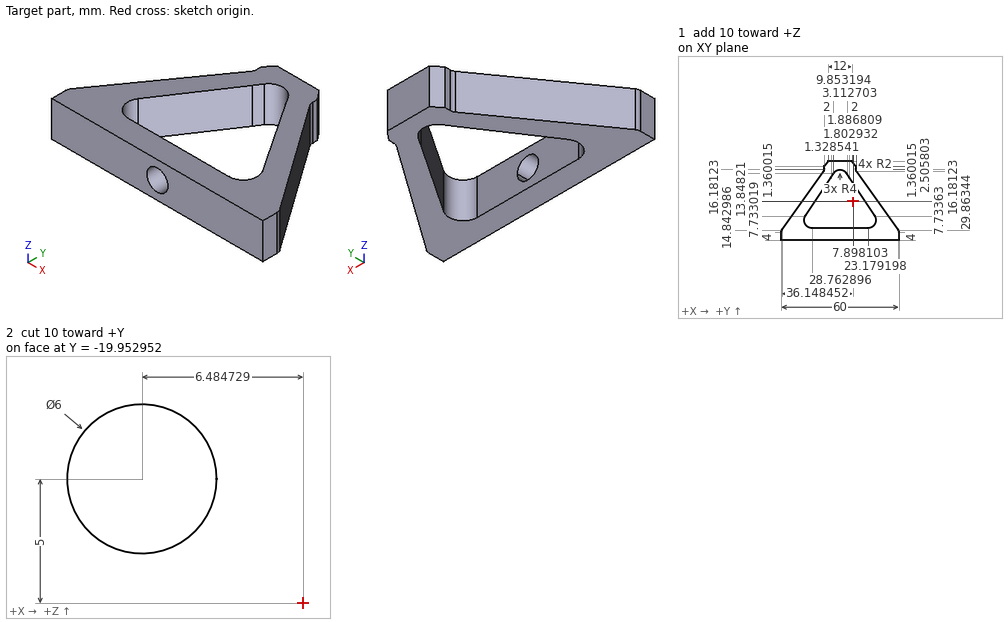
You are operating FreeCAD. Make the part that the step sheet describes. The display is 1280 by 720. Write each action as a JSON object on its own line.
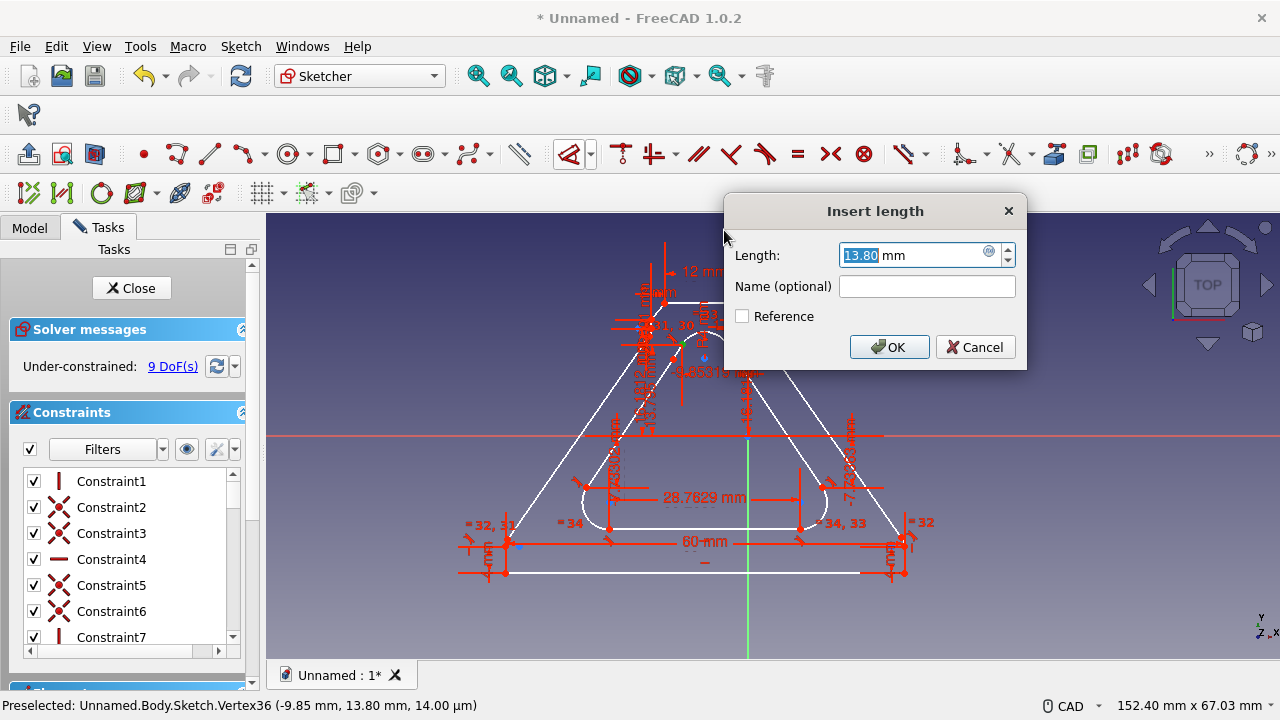
{"action": "type", "text": "13.84821"}
{"action": "key", "text": "Return"}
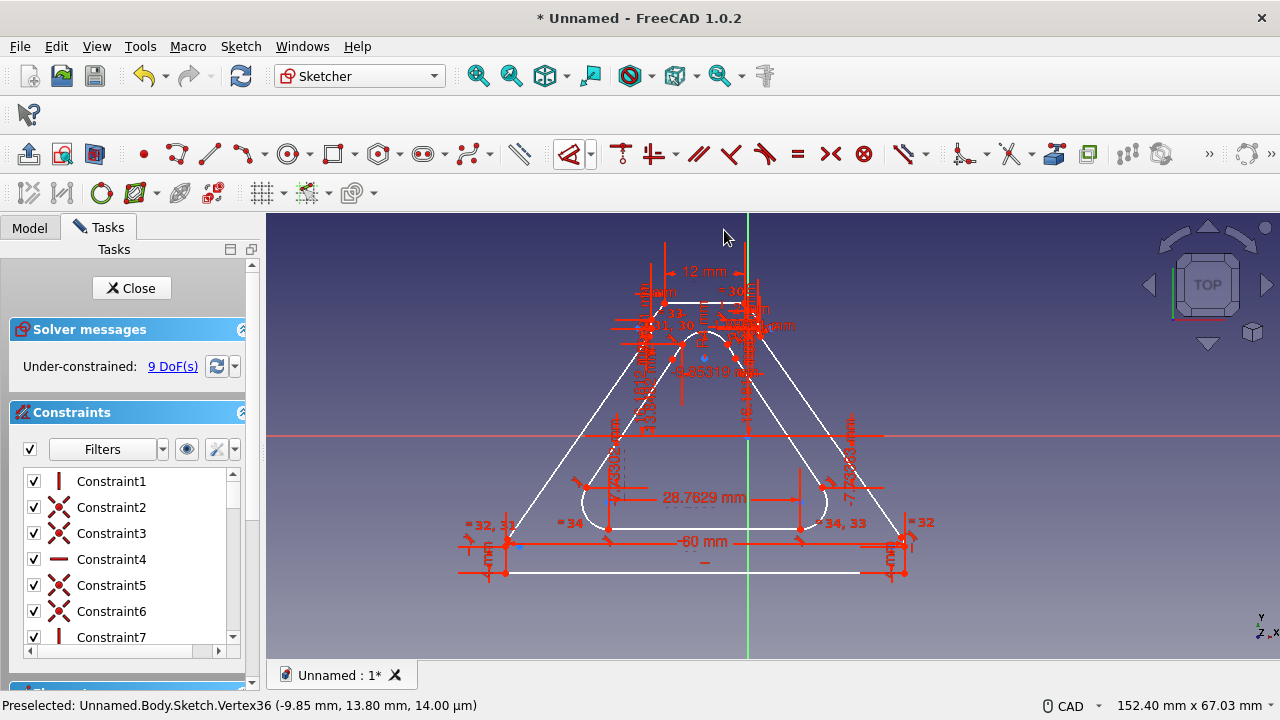
{"action": "scroll", "coordinate": [728, 345], "scroll_direction": "up", "scroll_amount": 4}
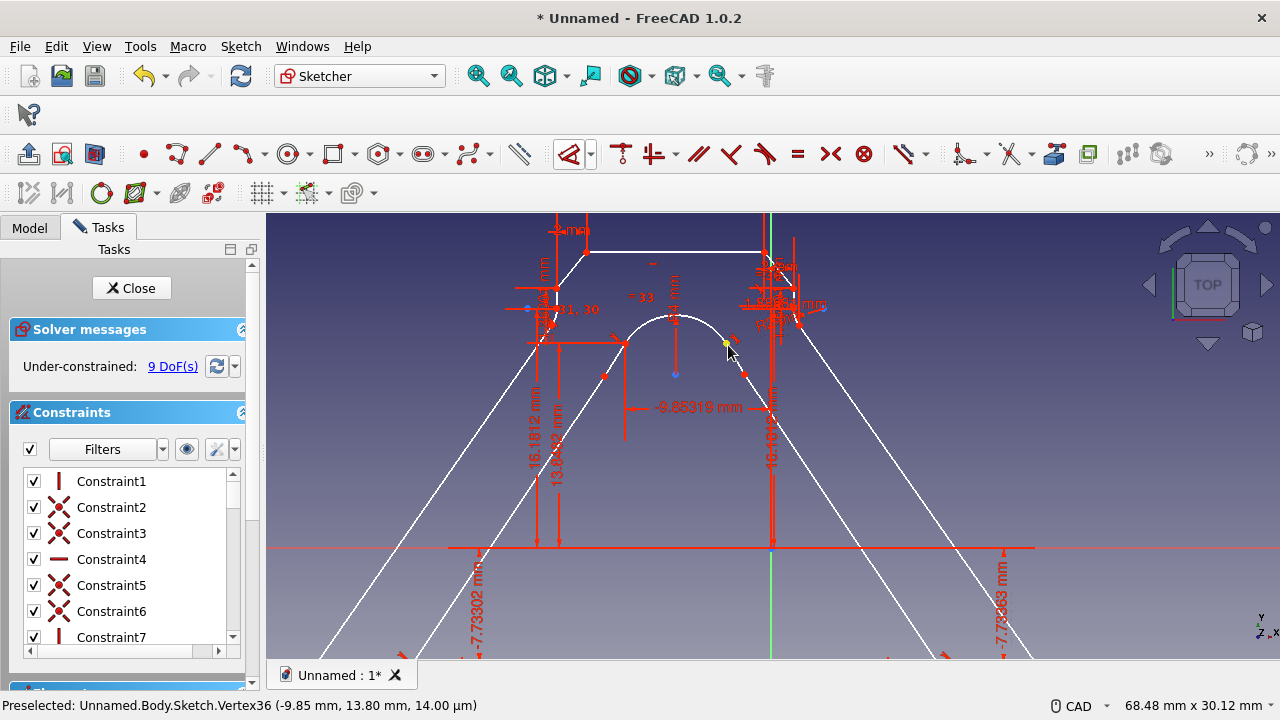
{"action": "left_click", "coordinate": [726, 344]}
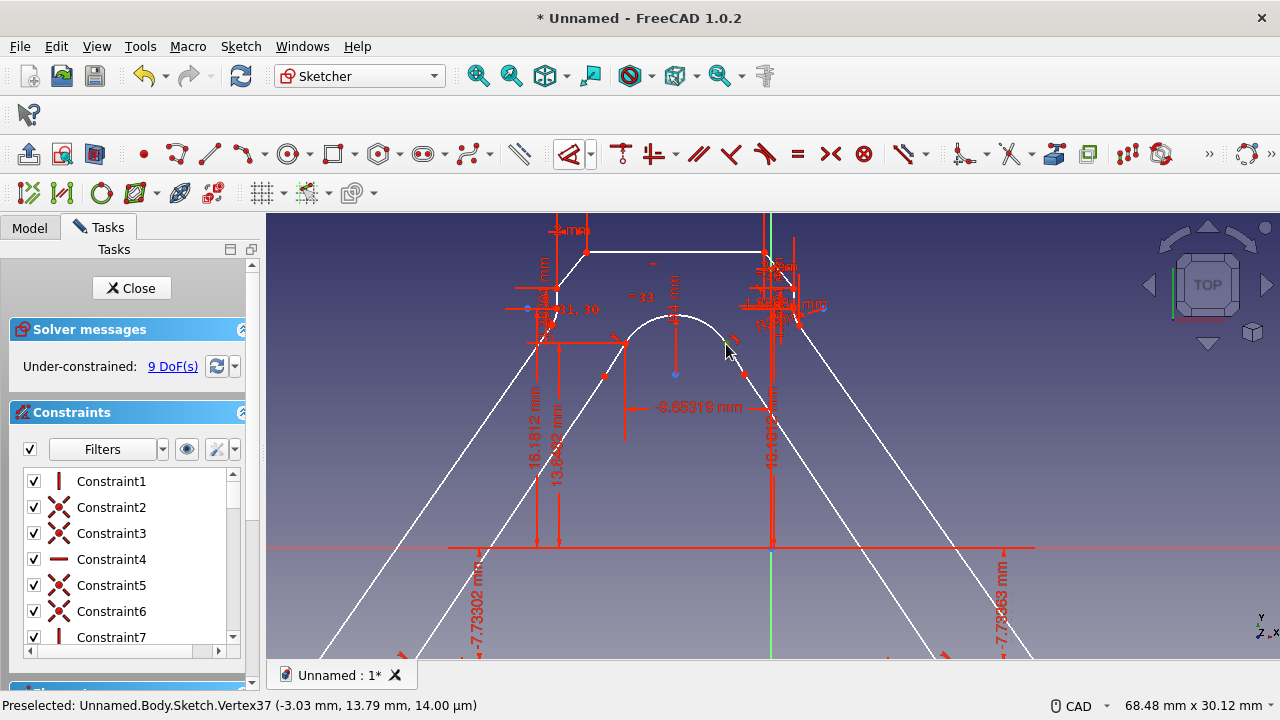
{"action": "left_click", "coordinate": [590, 154]}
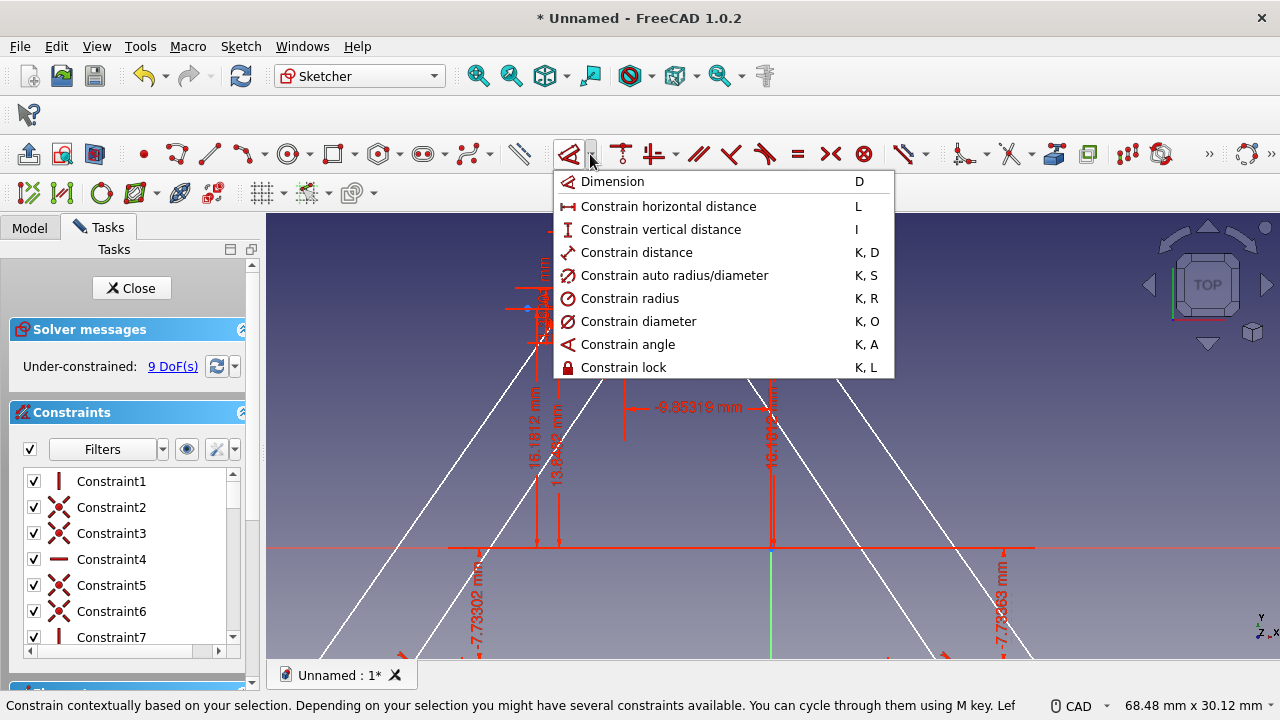
{"action": "left_click", "coordinate": [724, 206]}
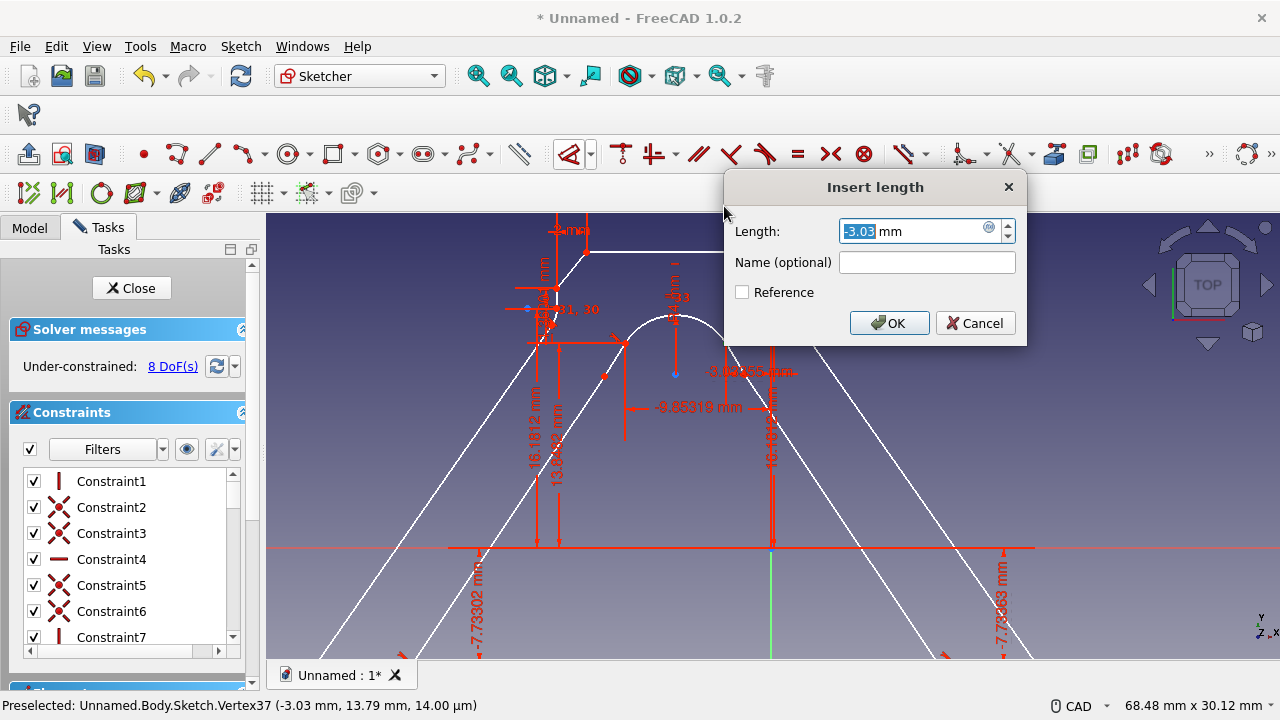
{"action": "type", "text": "-3.112703"}
{"action": "key", "text": "Return"}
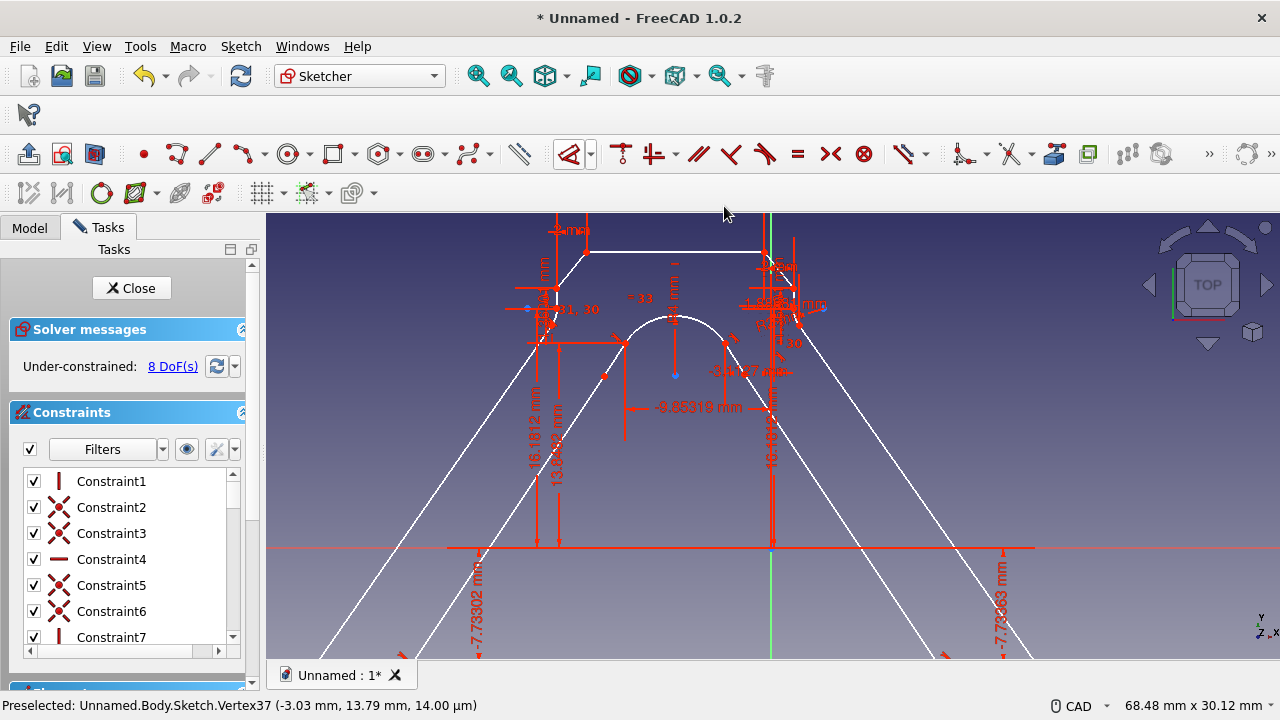
{"action": "scroll", "coordinate": [745, 374], "scroll_direction": "up", "scroll_amount": 2}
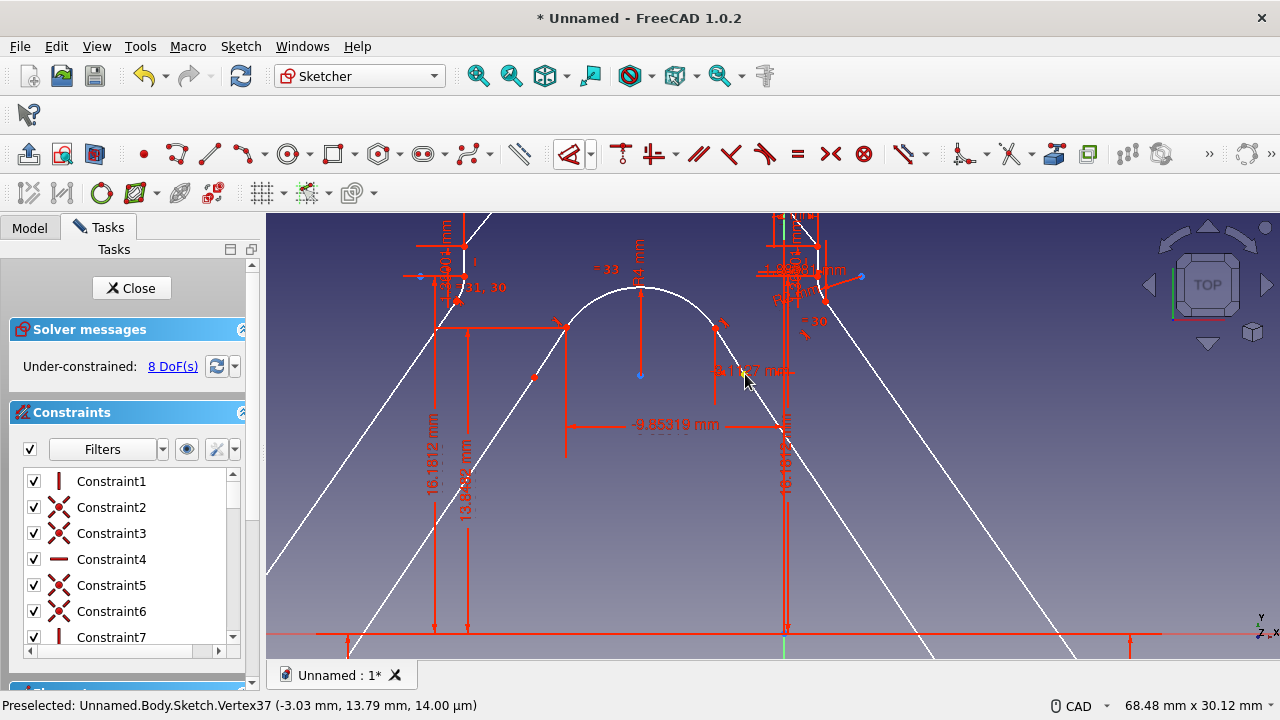
{"action": "left_click", "coordinate": [744, 375]}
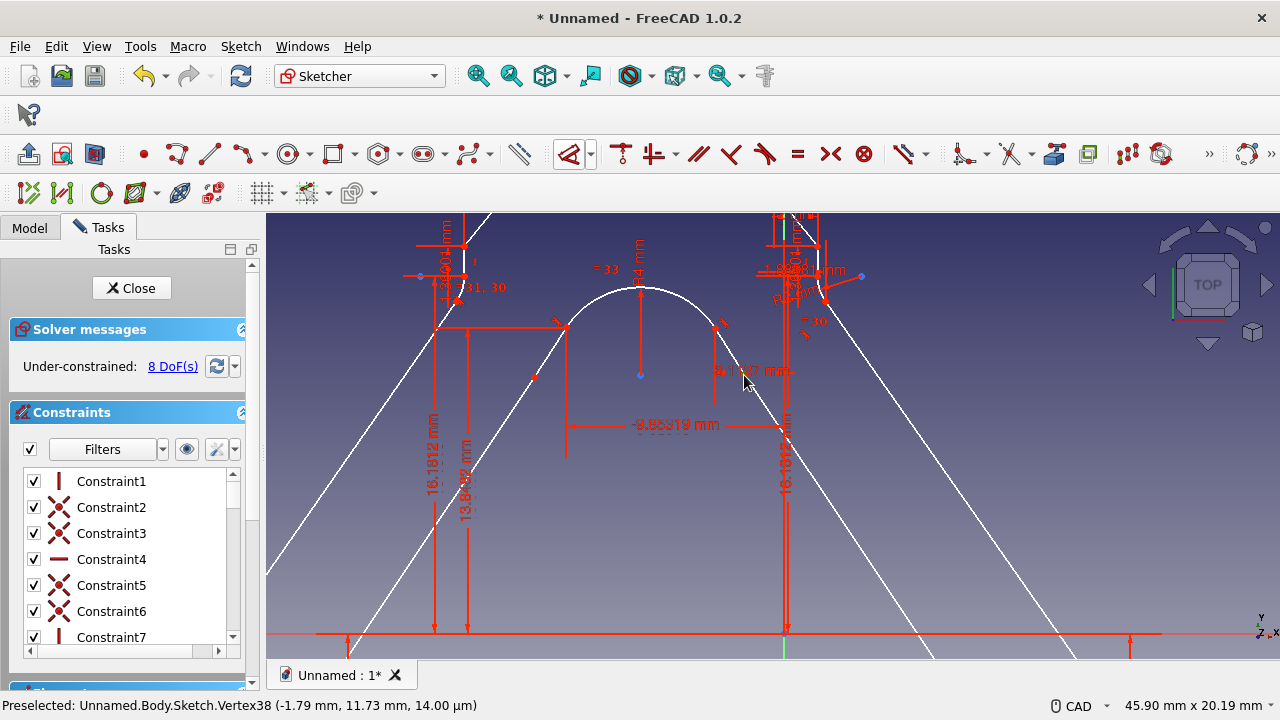
{"action": "left_click", "coordinate": [590, 154]}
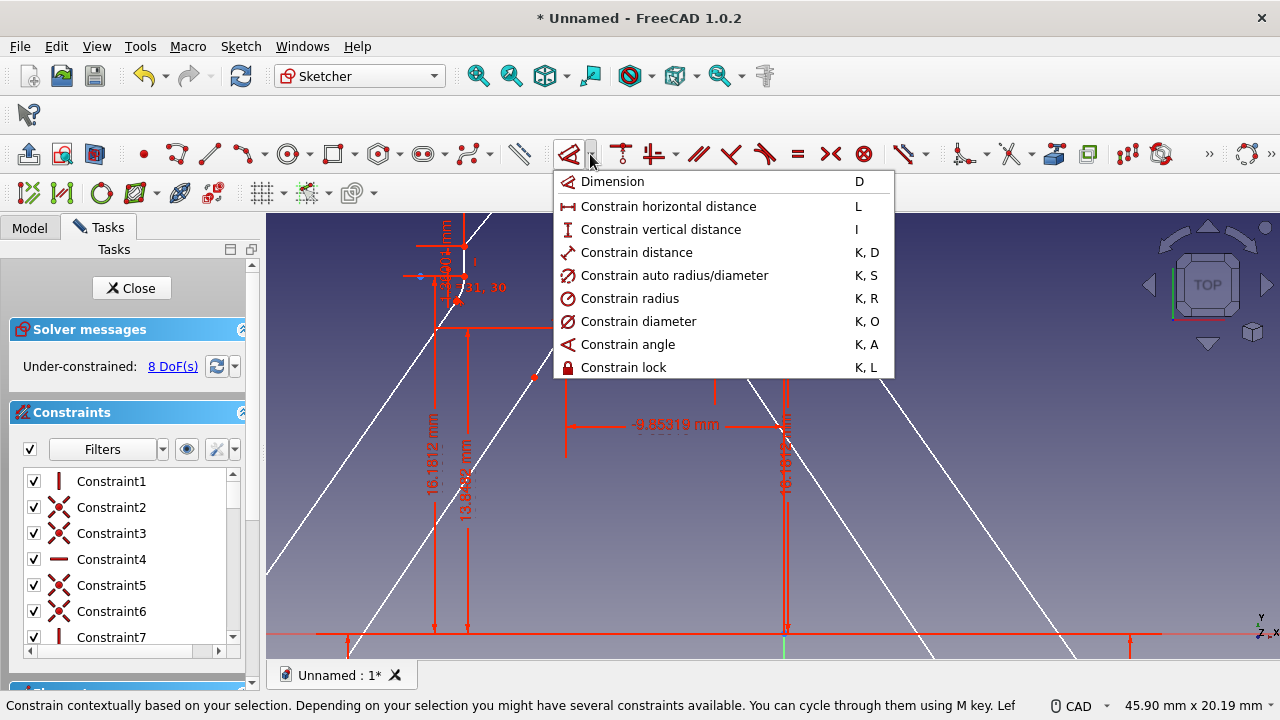
{"action": "left_click", "coordinate": [724, 206]}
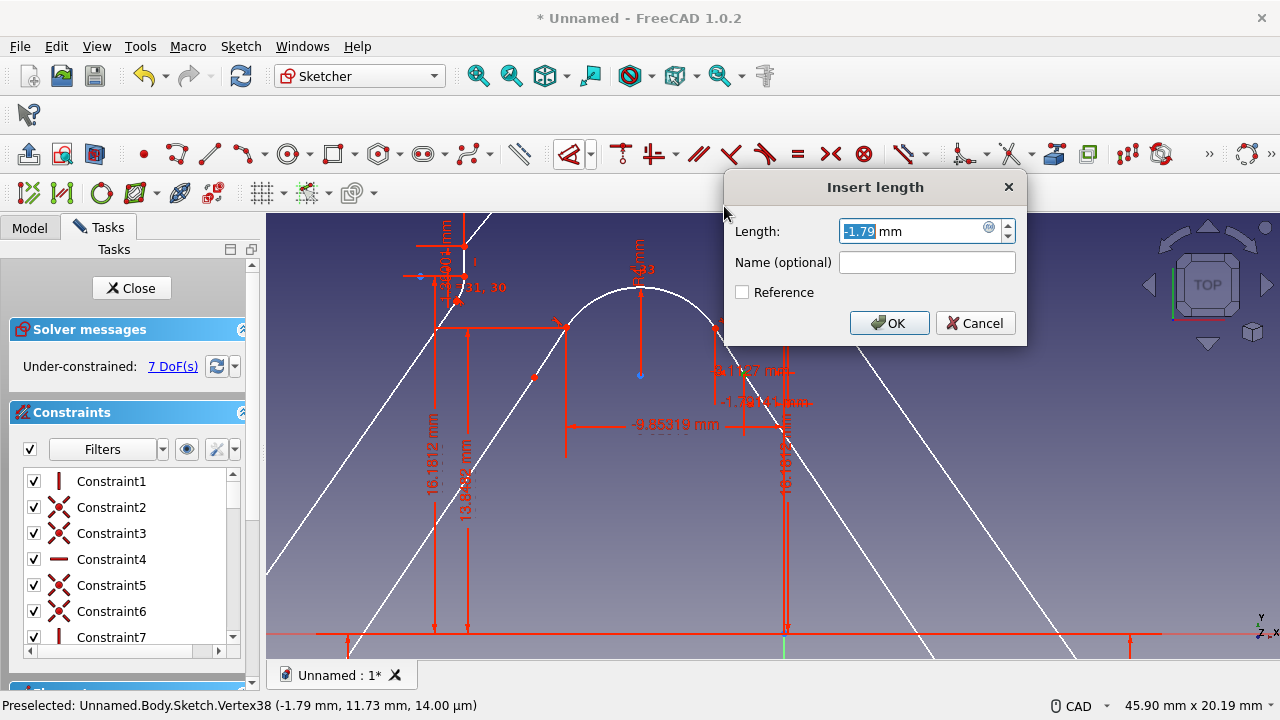
{"action": "type", "text": "-1.802932"}
{"action": "key", "text": "Return"}